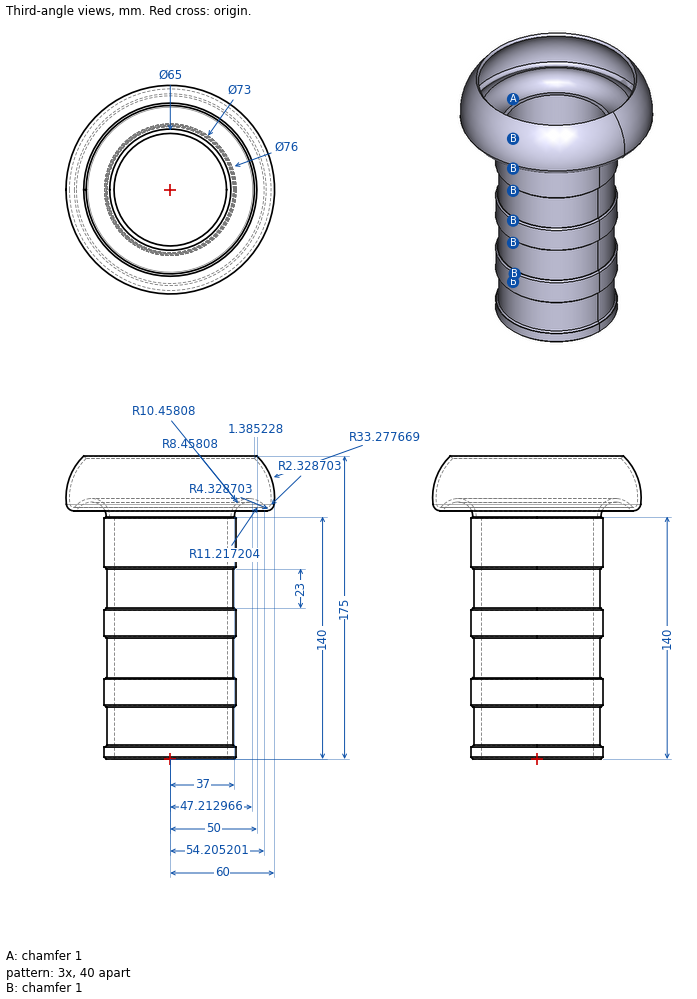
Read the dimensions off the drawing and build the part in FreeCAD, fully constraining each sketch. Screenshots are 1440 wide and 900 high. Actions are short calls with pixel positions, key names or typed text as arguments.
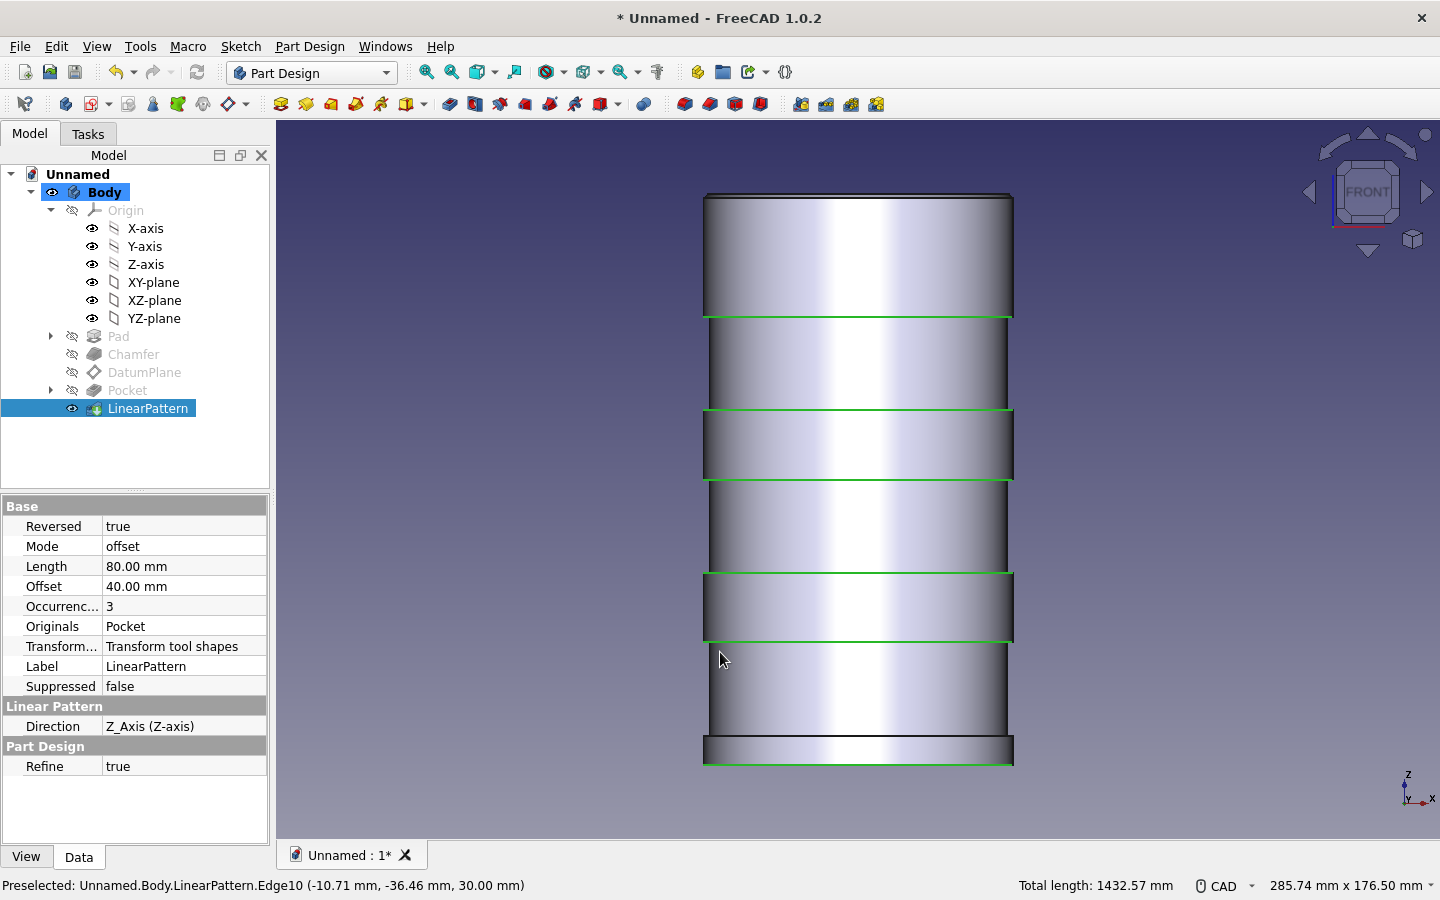
key(3)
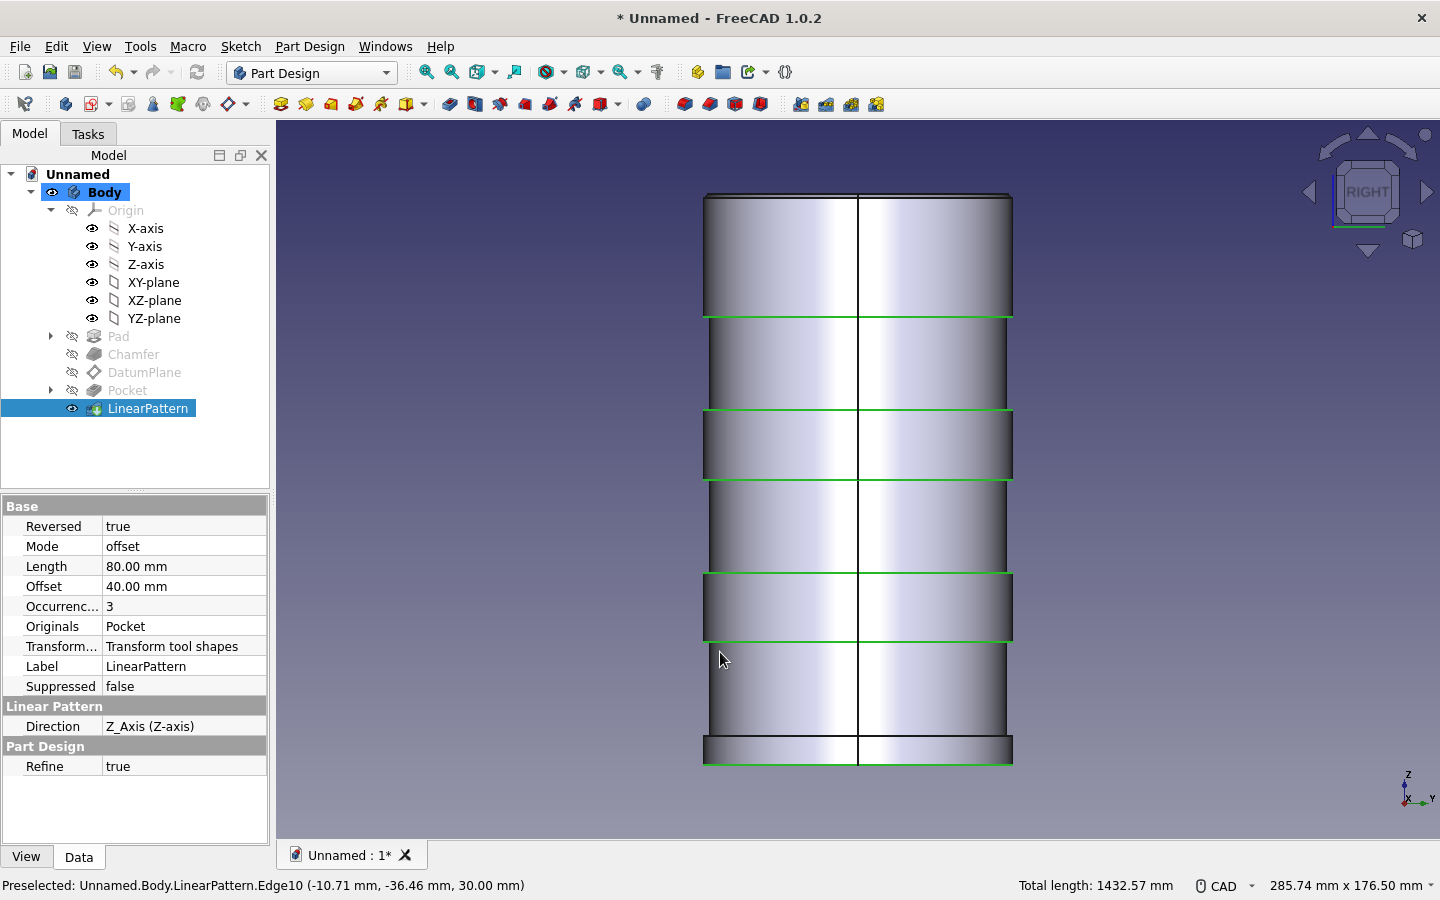
key(5)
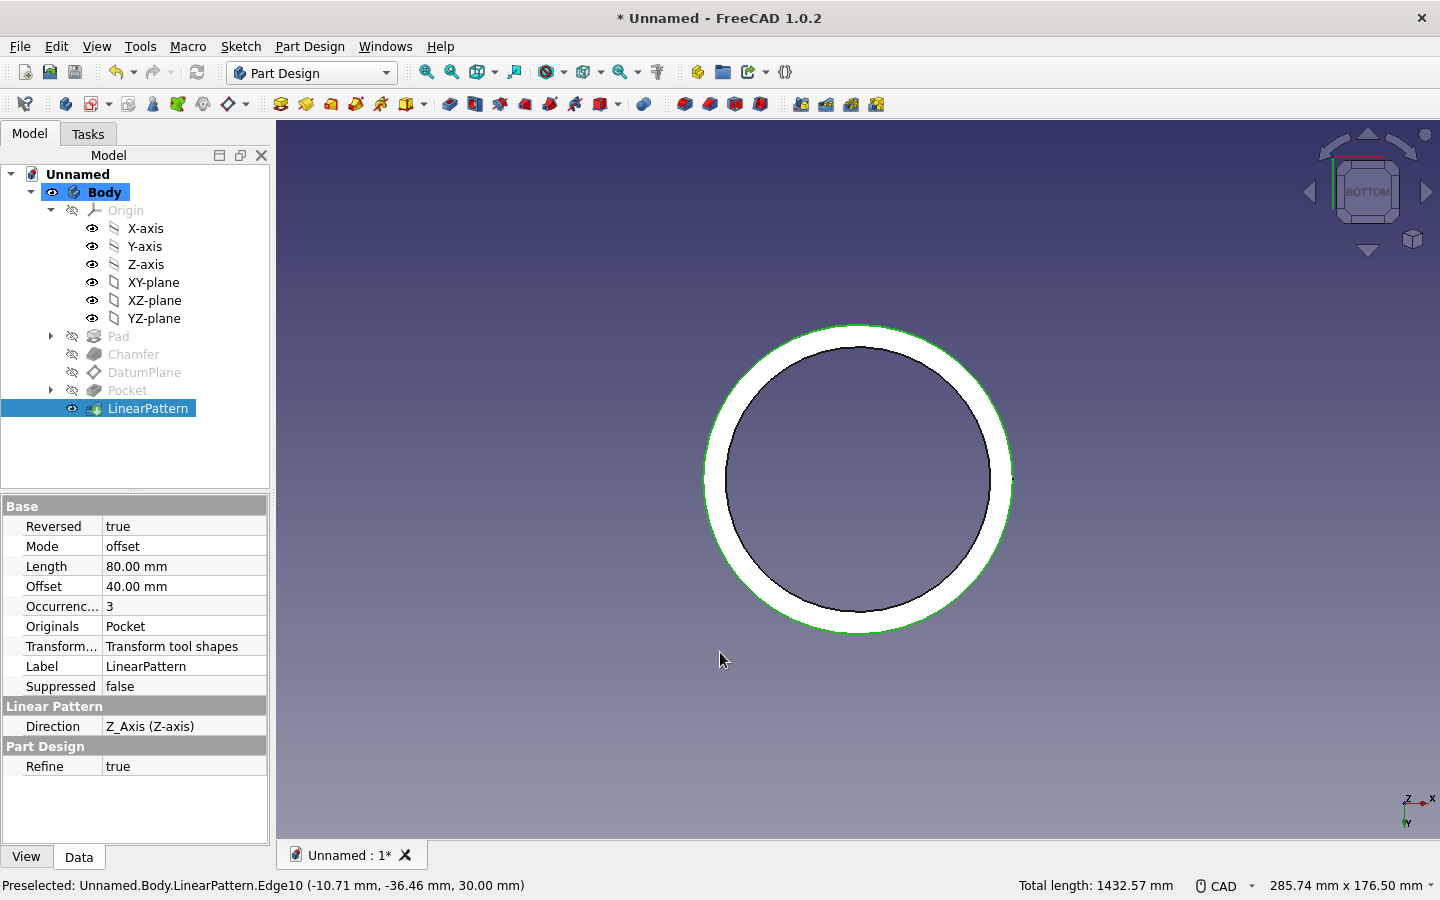
click(427, 72)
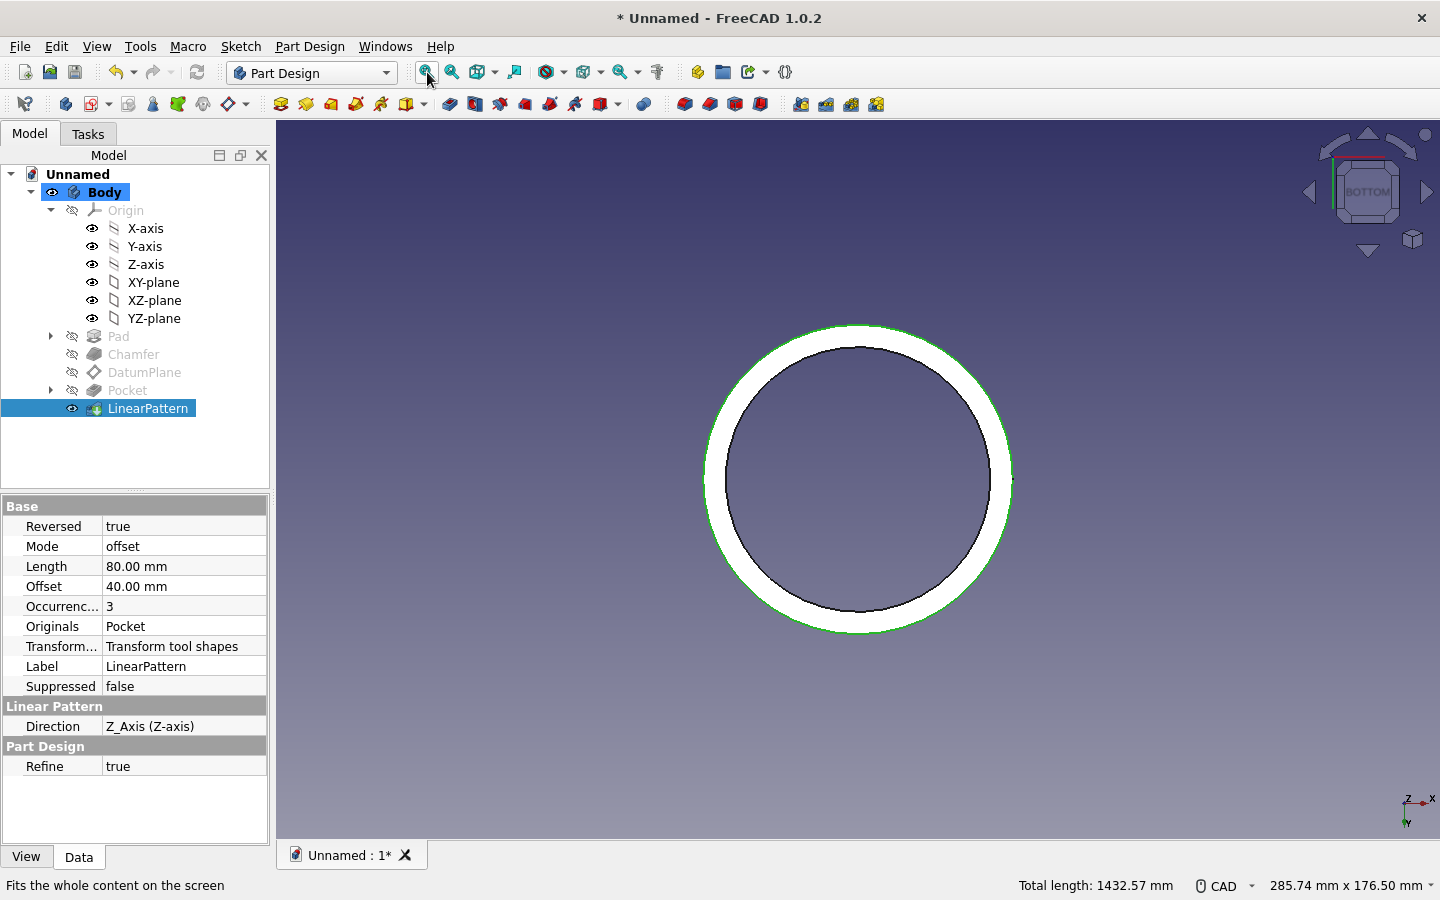
key(4)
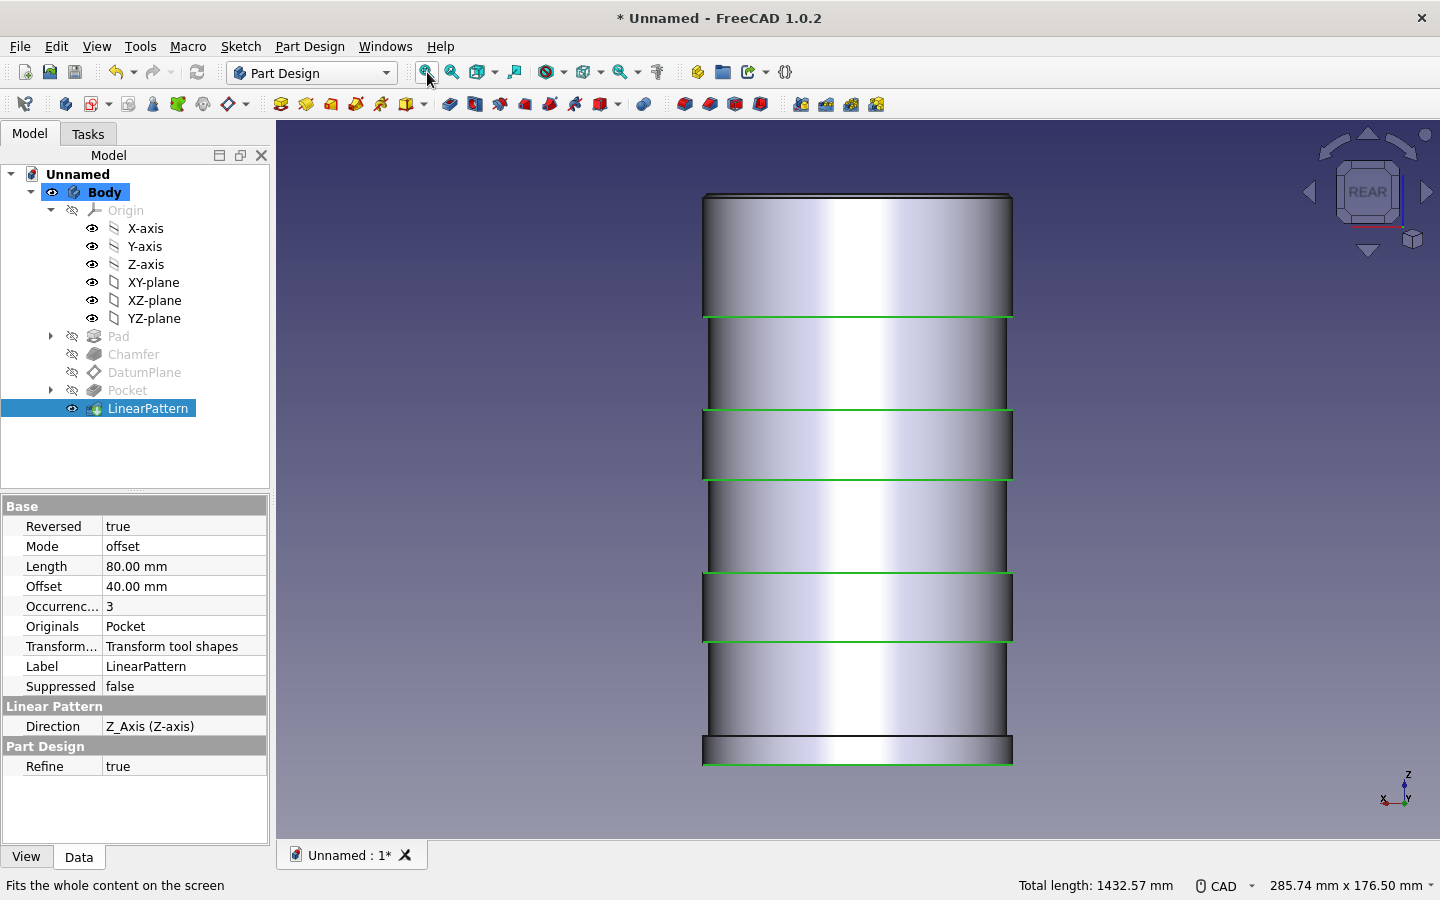
key(6)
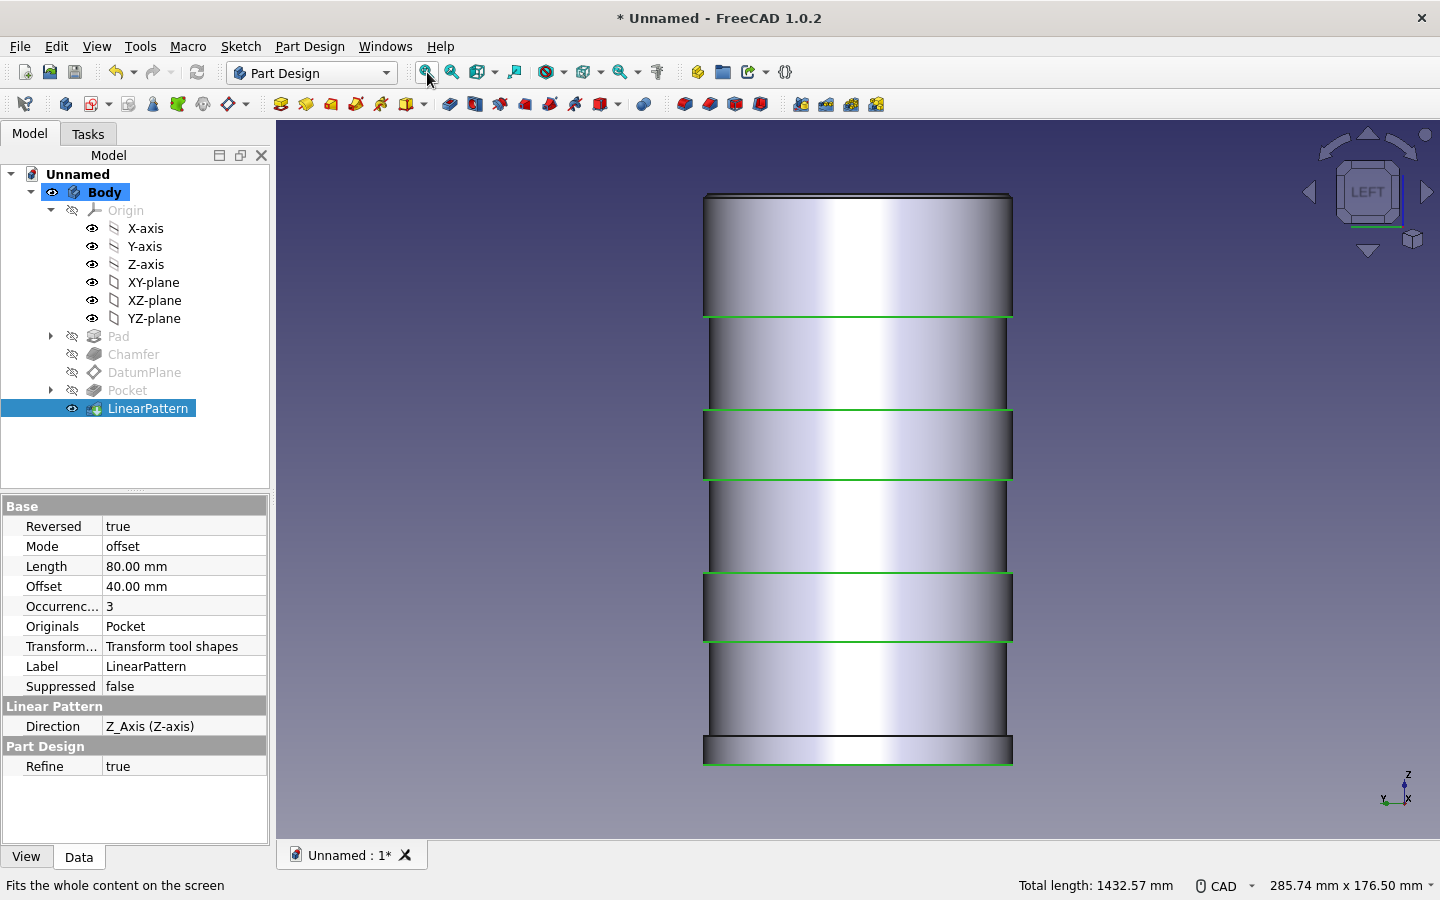
key(v)
key(3)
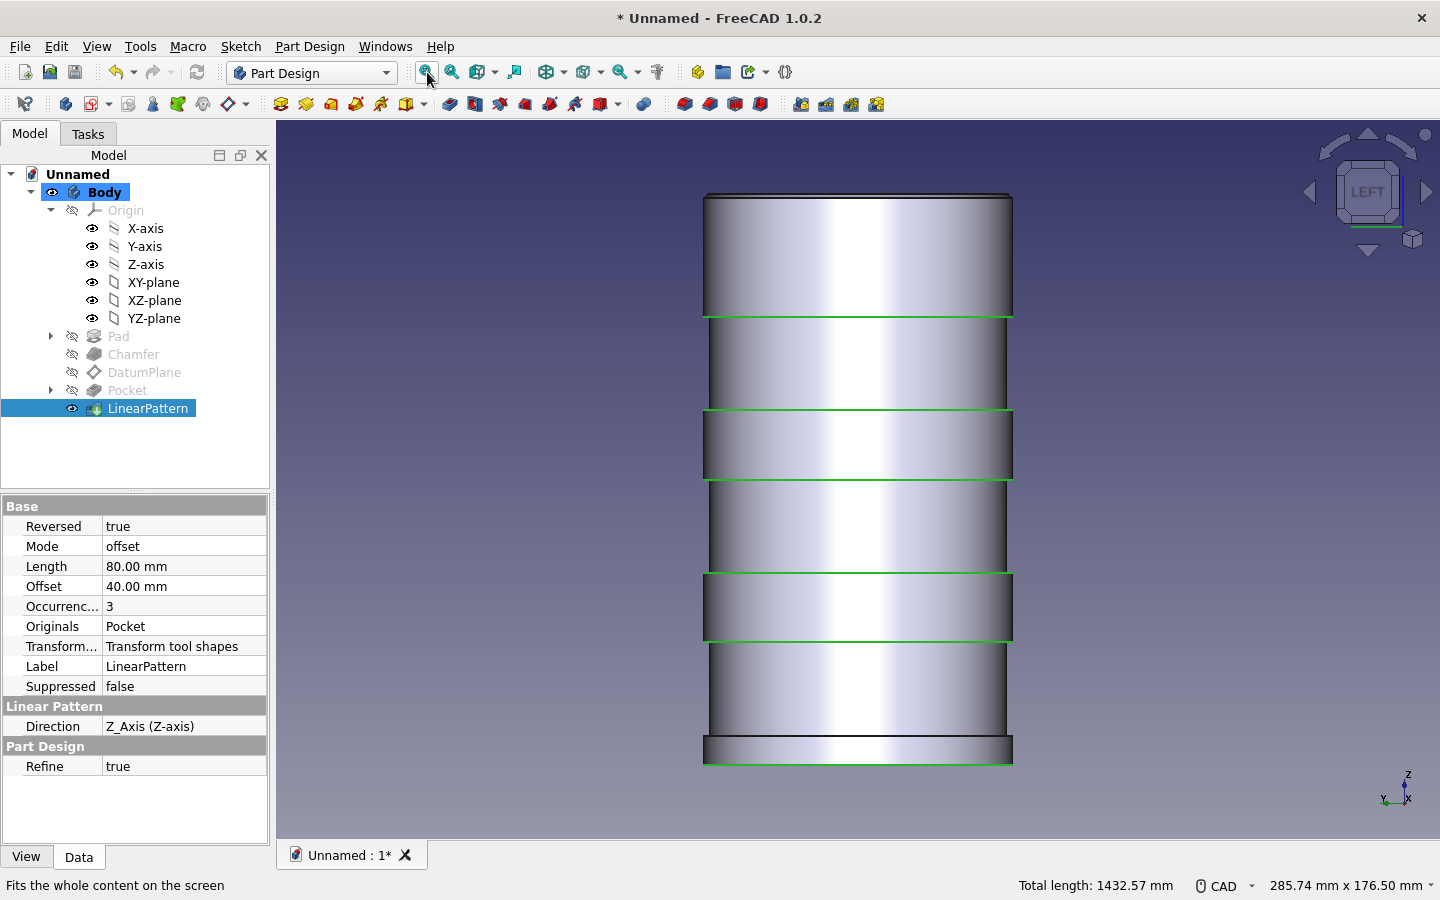
key(0)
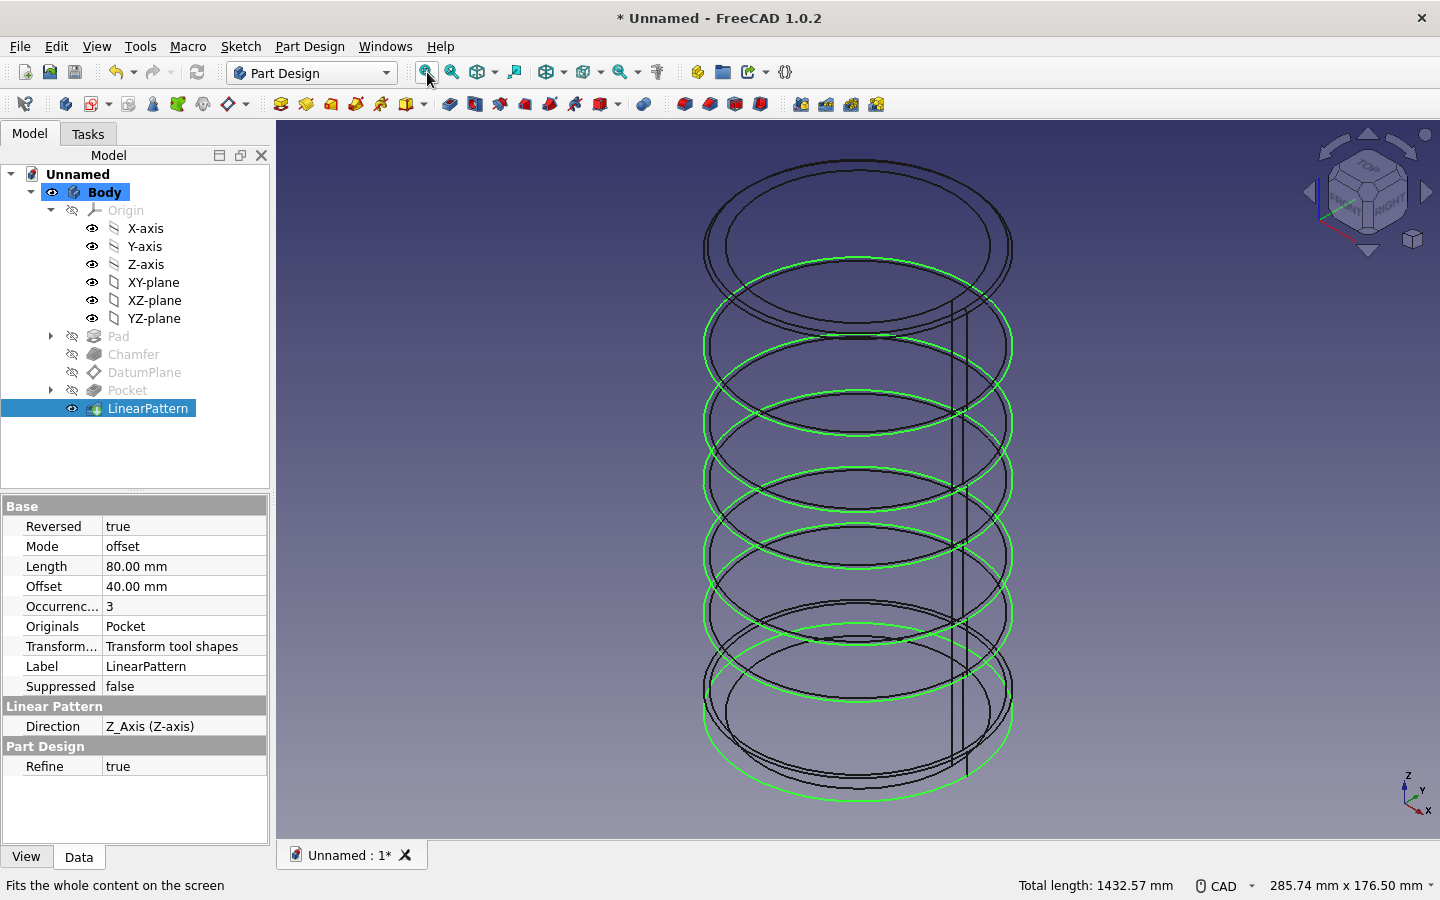
click(427, 72)